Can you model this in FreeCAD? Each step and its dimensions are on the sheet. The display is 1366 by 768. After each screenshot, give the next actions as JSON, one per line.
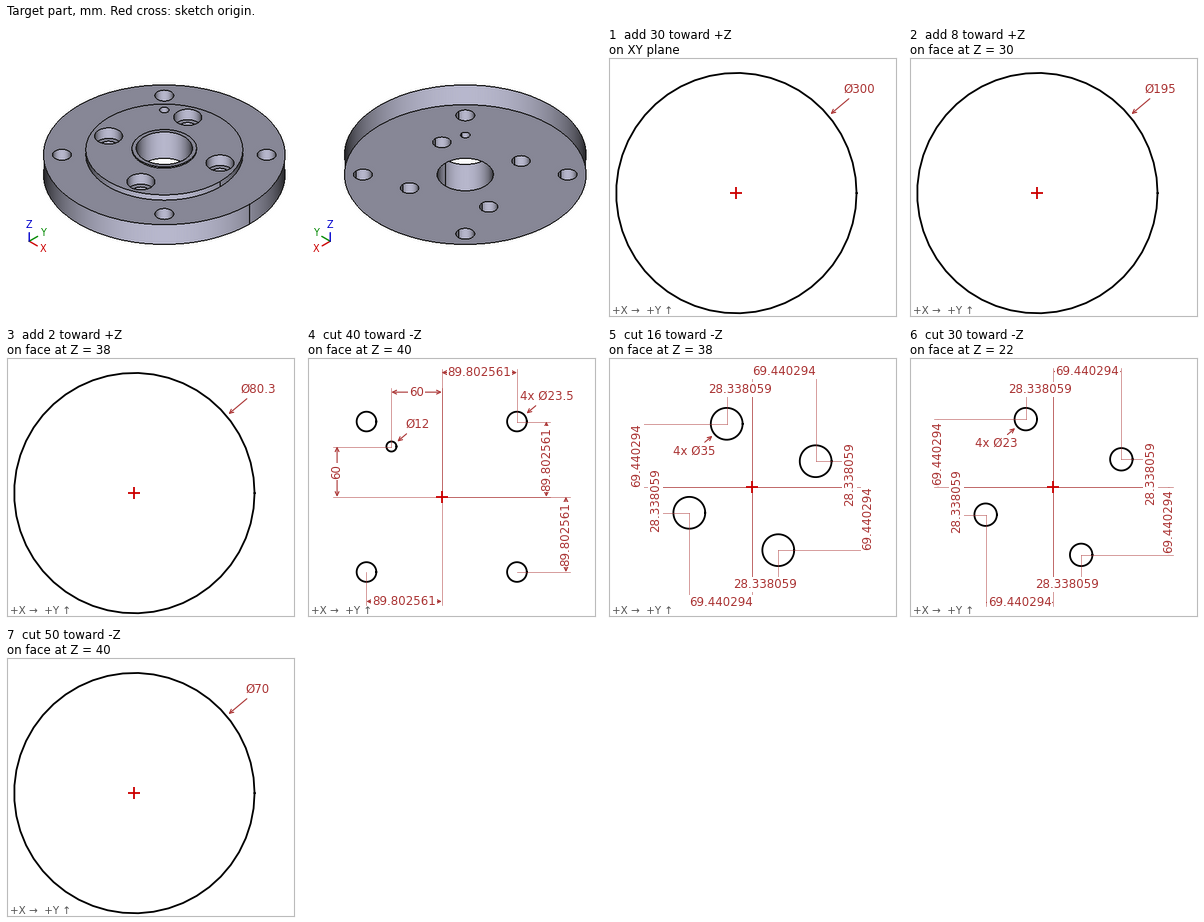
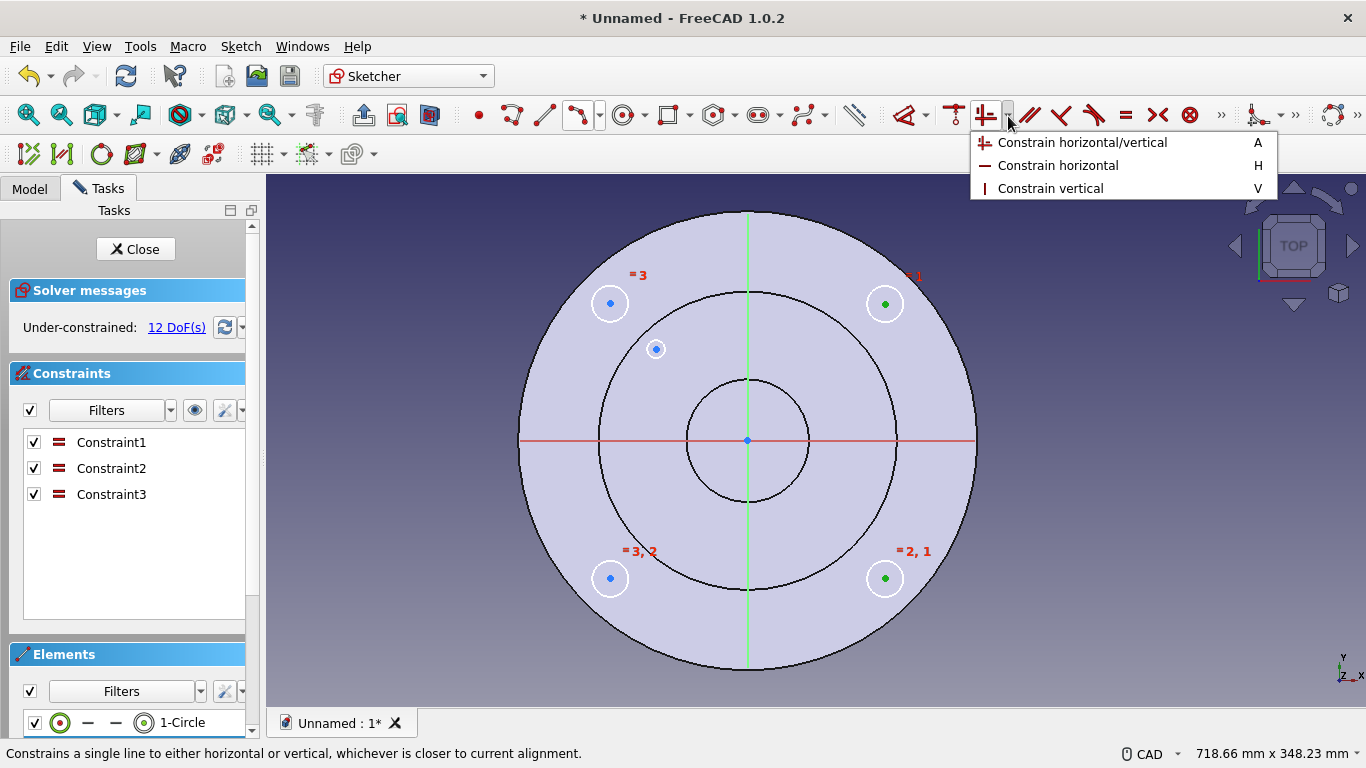
{"action": "left_click", "coordinate": [1124, 188]}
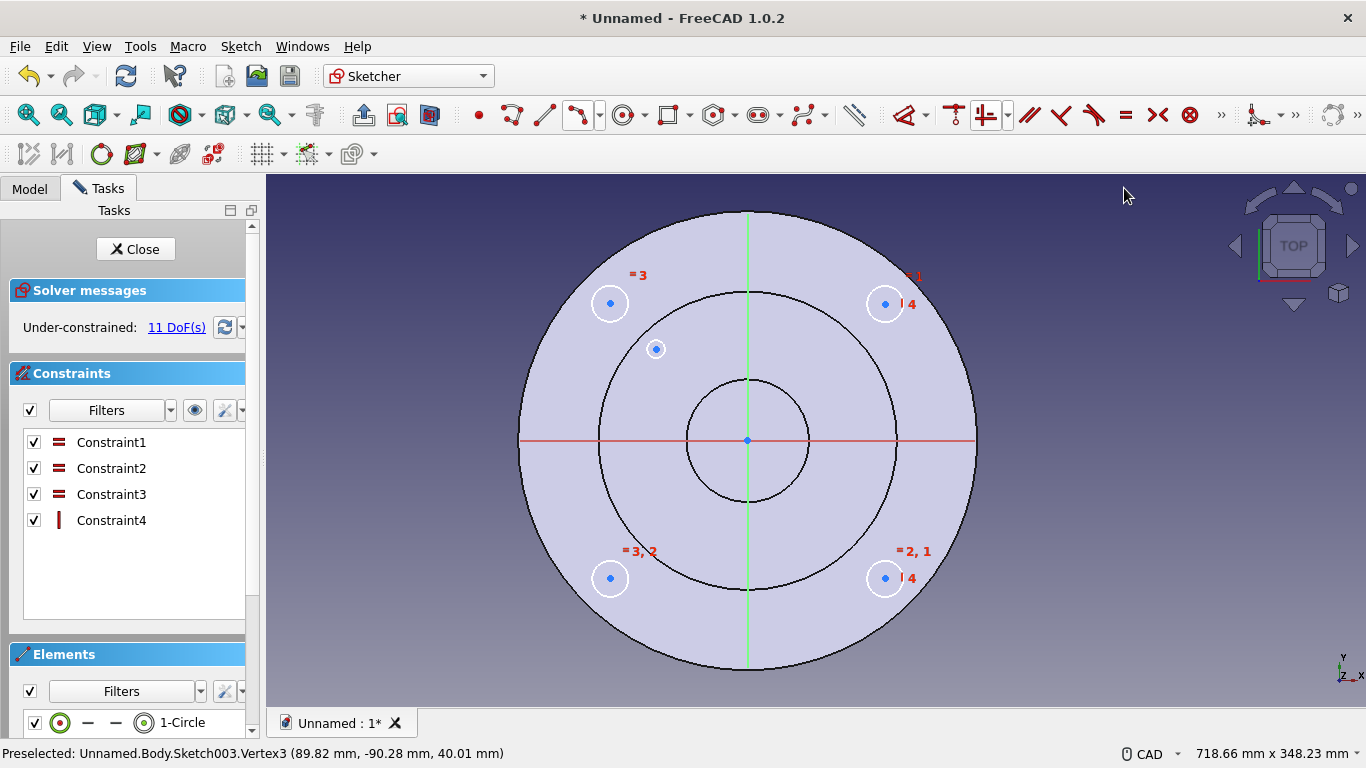
{"action": "left_click", "coordinate": [885, 579]}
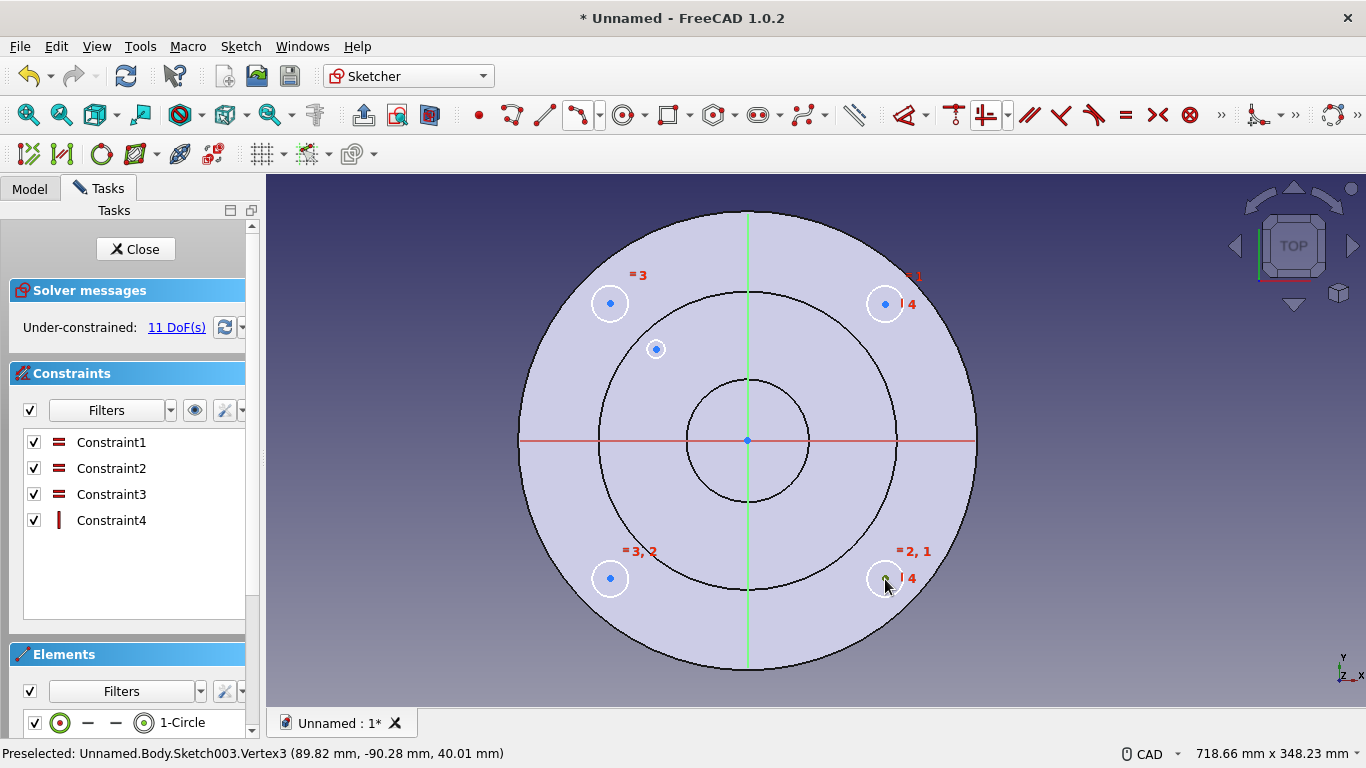
{"action": "left_click", "coordinate": [610, 579]}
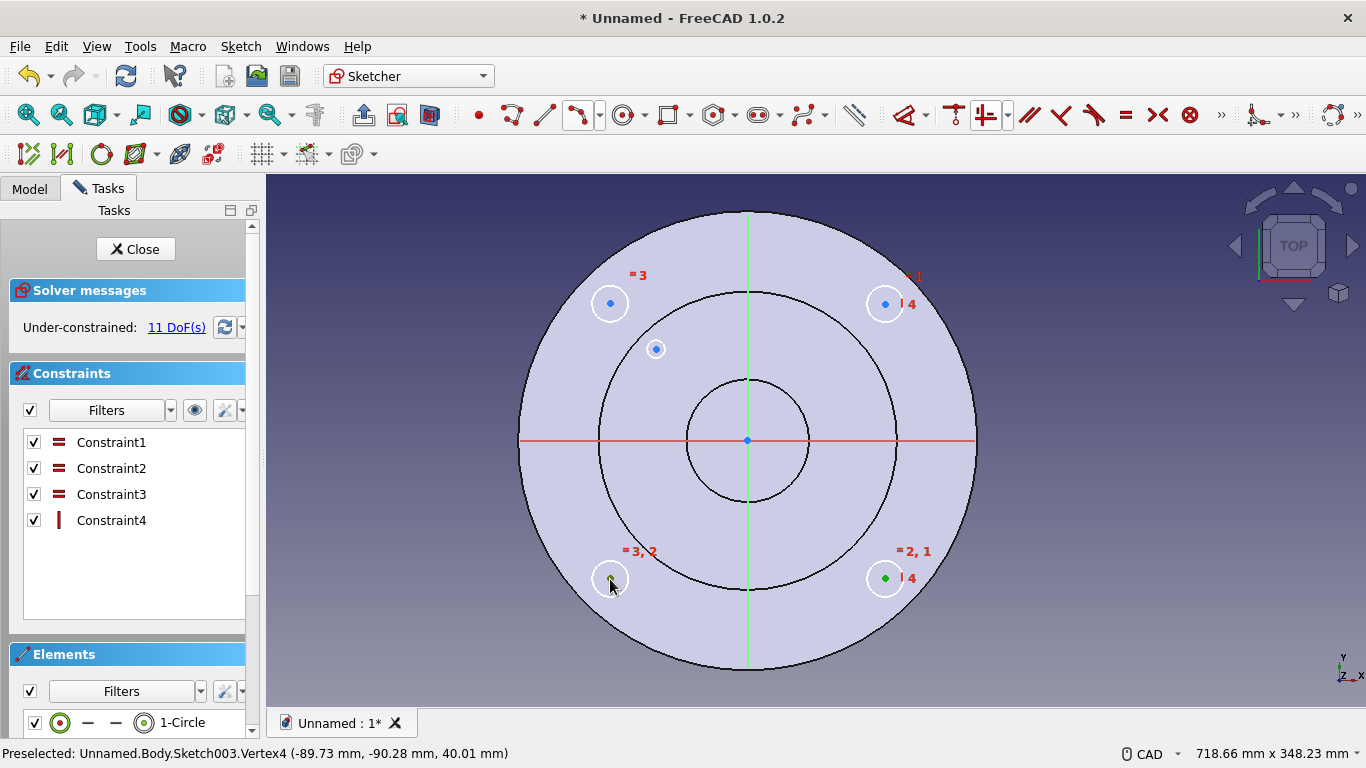
{"action": "key", "text": "h"}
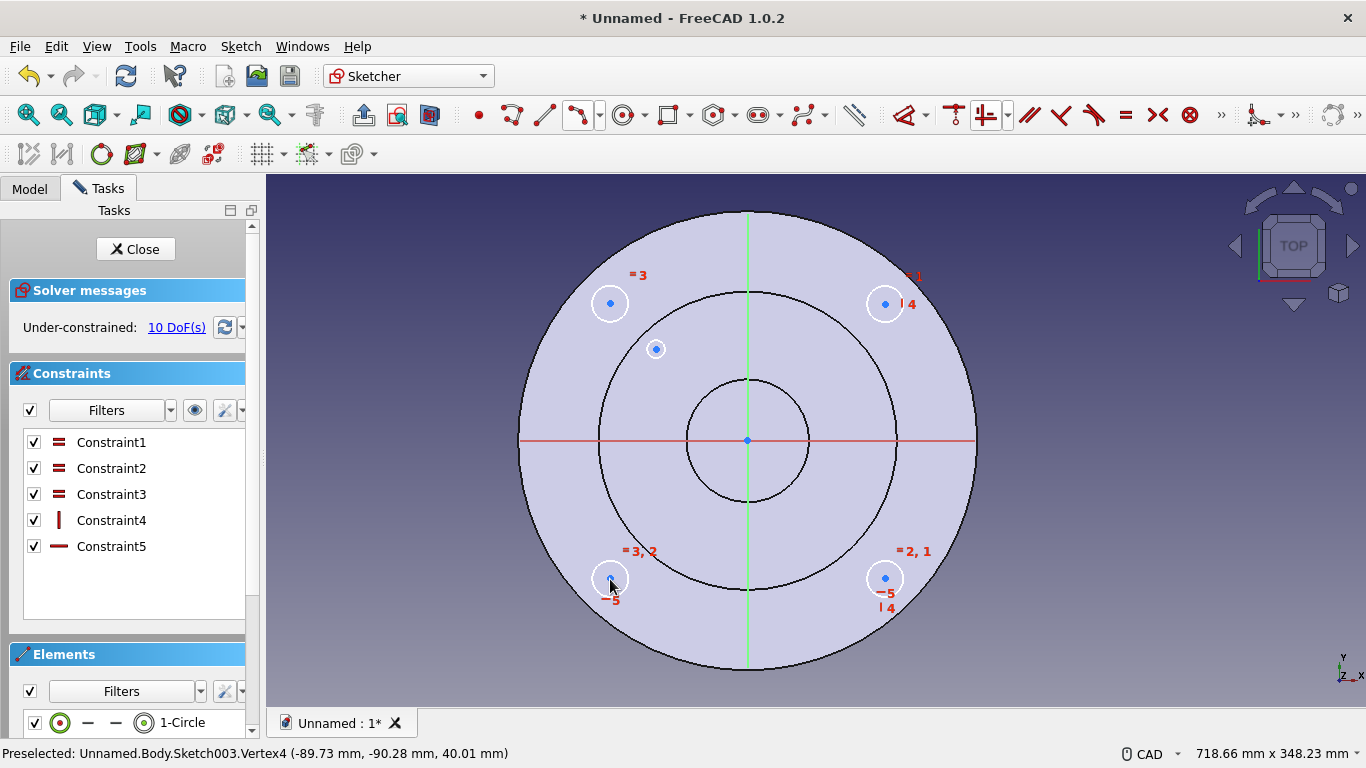
{"action": "left_click", "coordinate": [610, 579]}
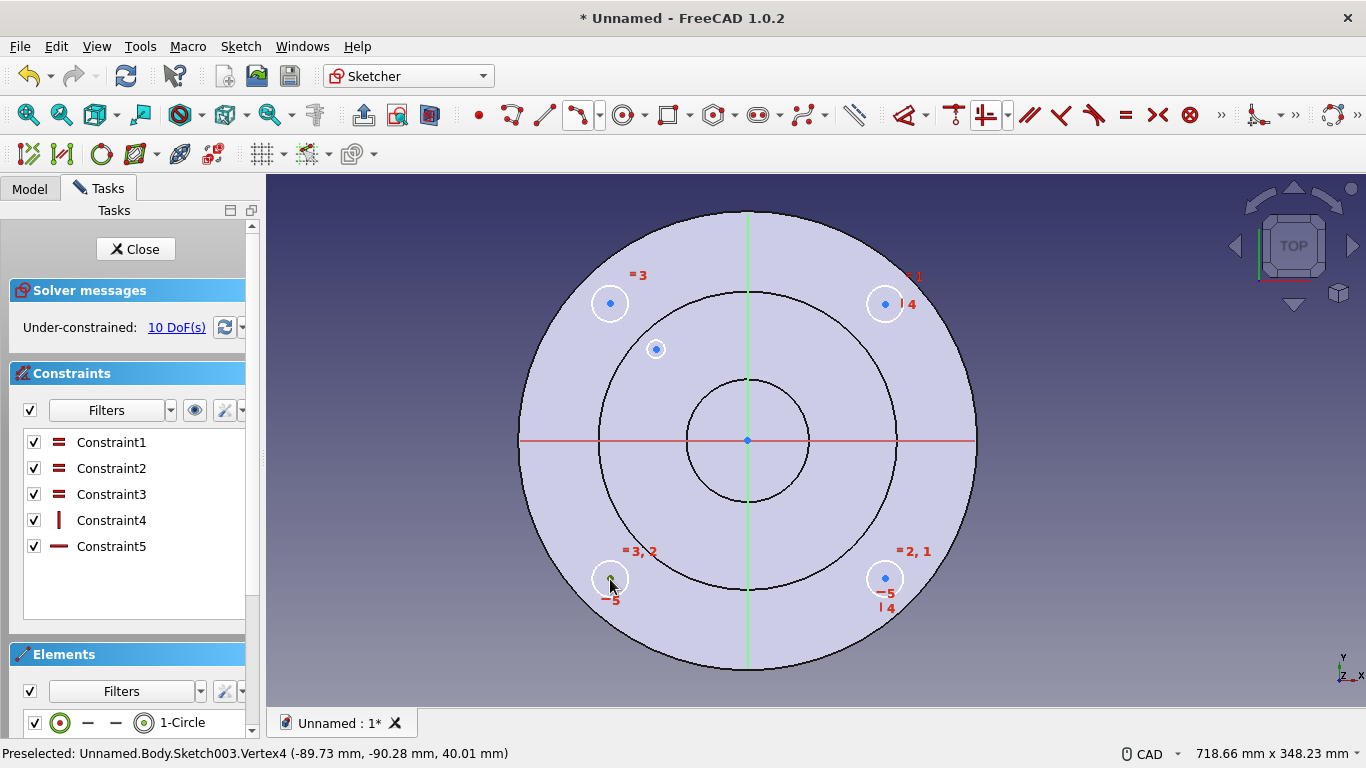
{"action": "left_click", "coordinate": [610, 304]}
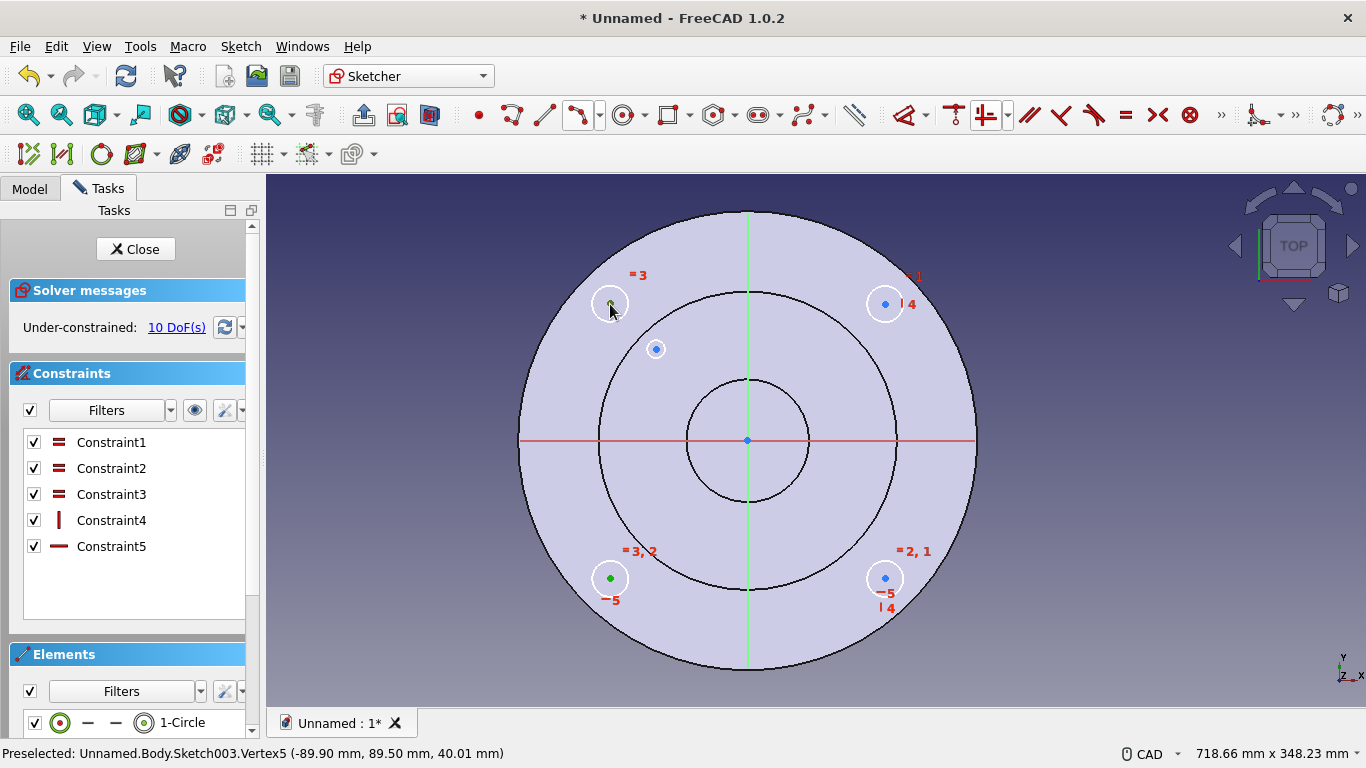
{"action": "key", "text": "v"}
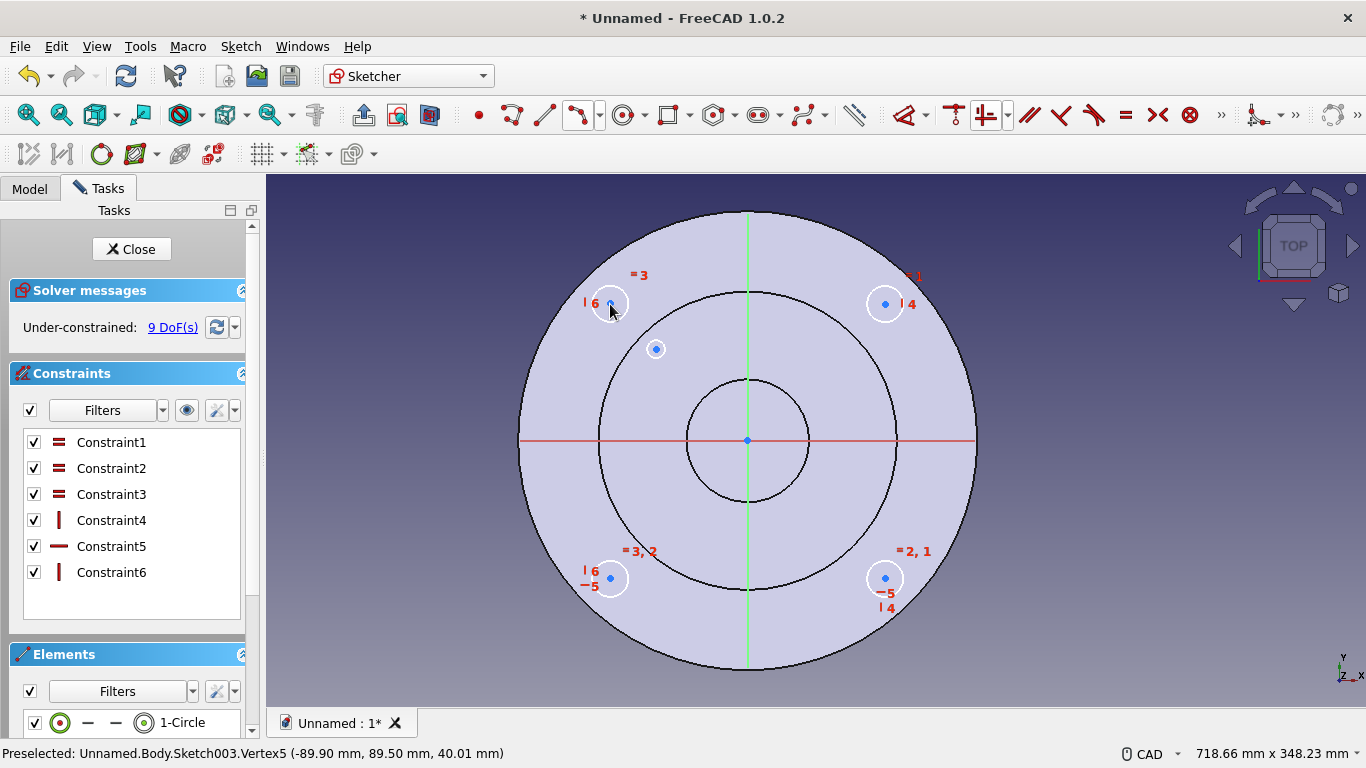
{"action": "left_click", "coordinate": [885, 304]}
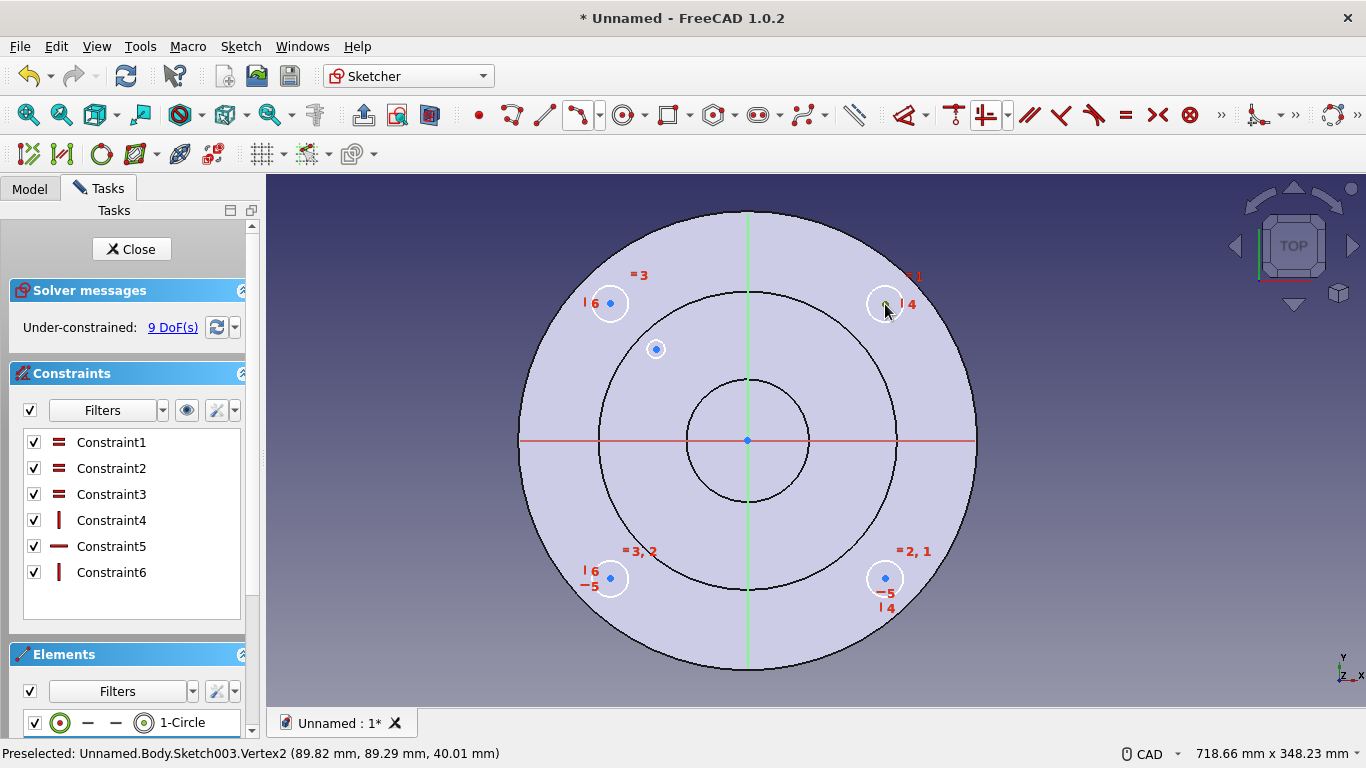
{"action": "left_click", "coordinate": [610, 304]}